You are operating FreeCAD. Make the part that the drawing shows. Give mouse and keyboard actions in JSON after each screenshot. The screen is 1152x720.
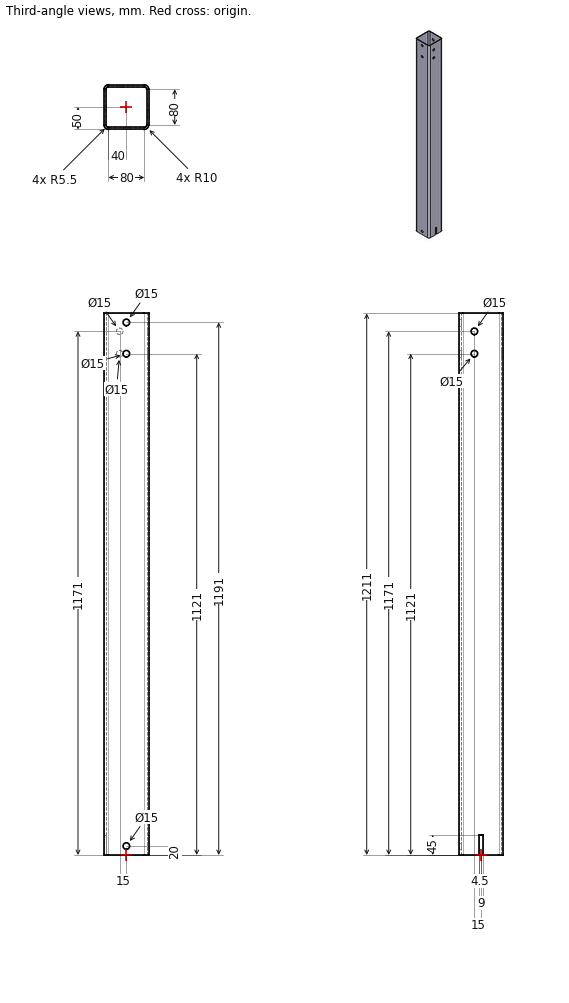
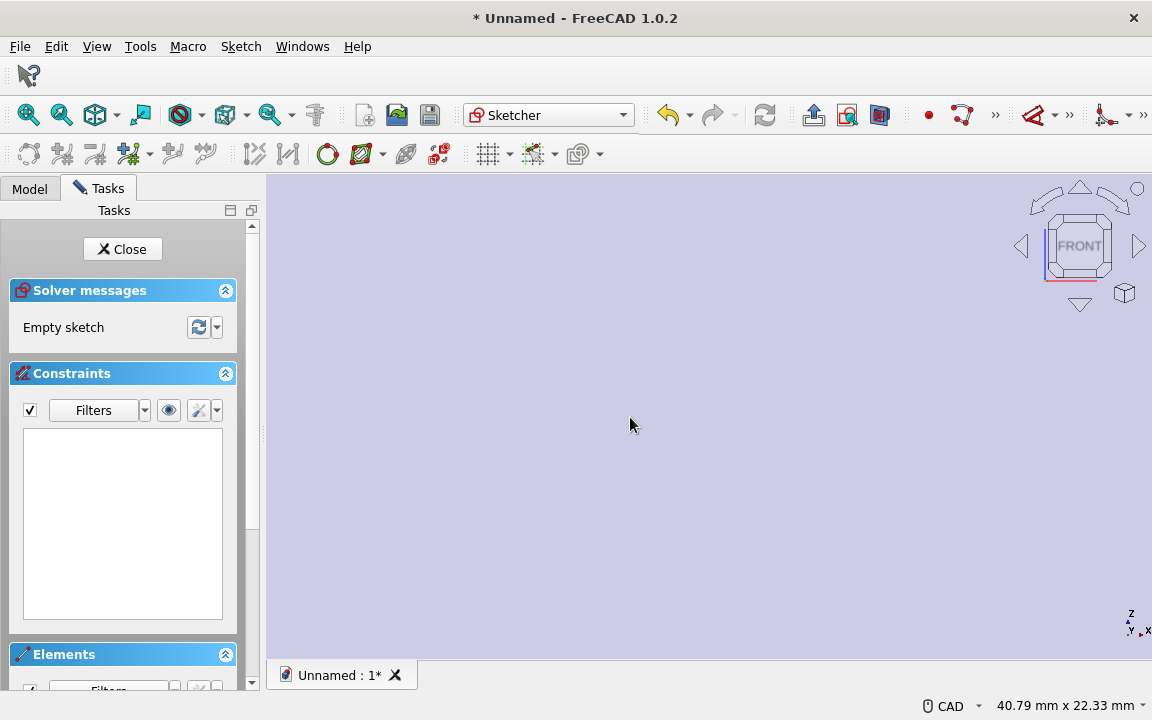
{"action": "key", "text": "g c"}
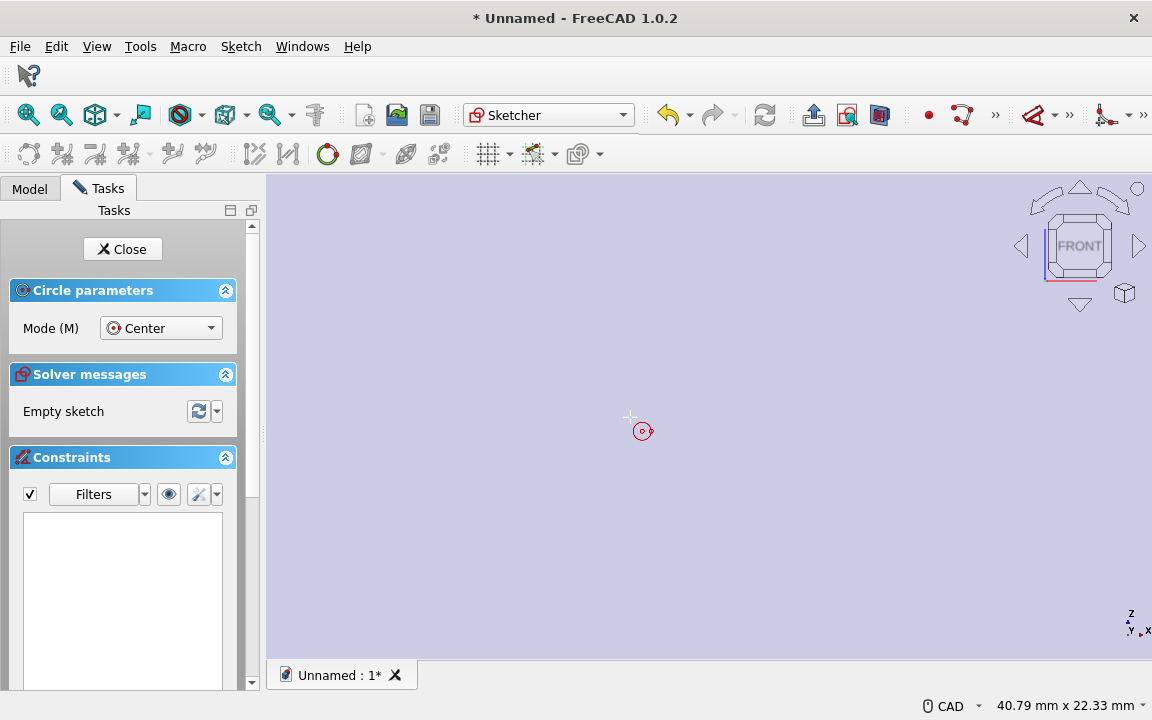
{"action": "left_click", "coordinate": [637, 412]}
{"action": "left_click", "coordinate": [752, 297]}
{"action": "key", "text": "Escape"}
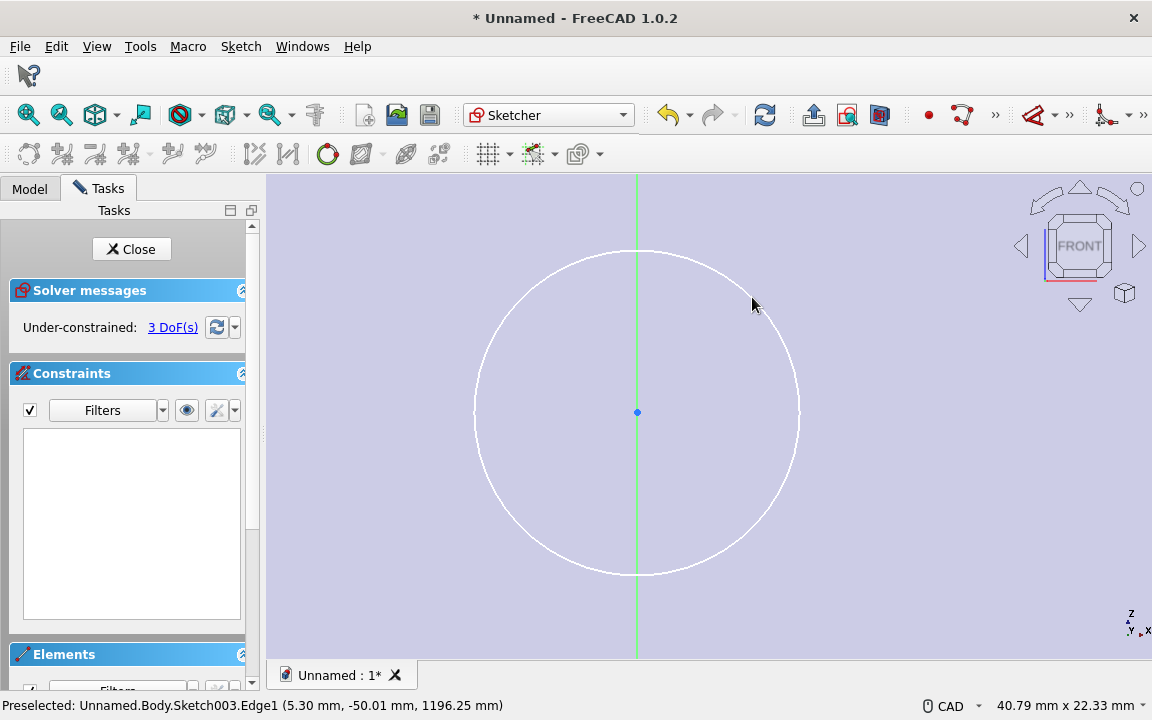
{"action": "left_click", "coordinate": [637, 413]}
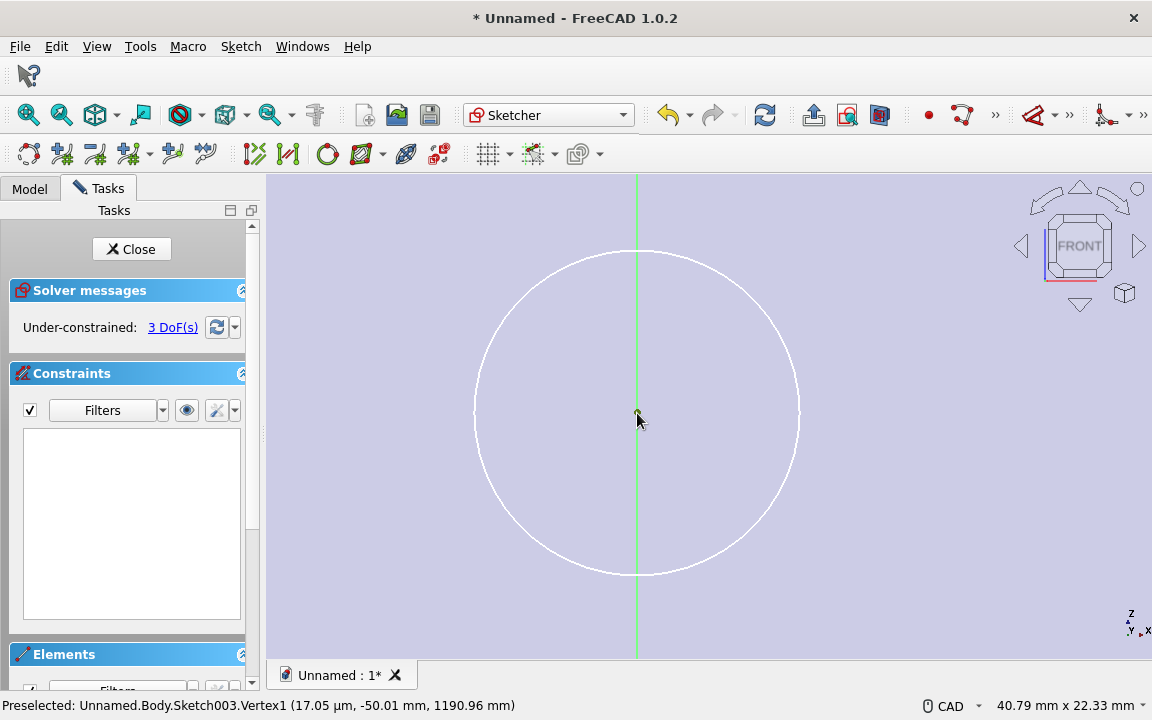
{"action": "left_click", "coordinate": [637, 539]}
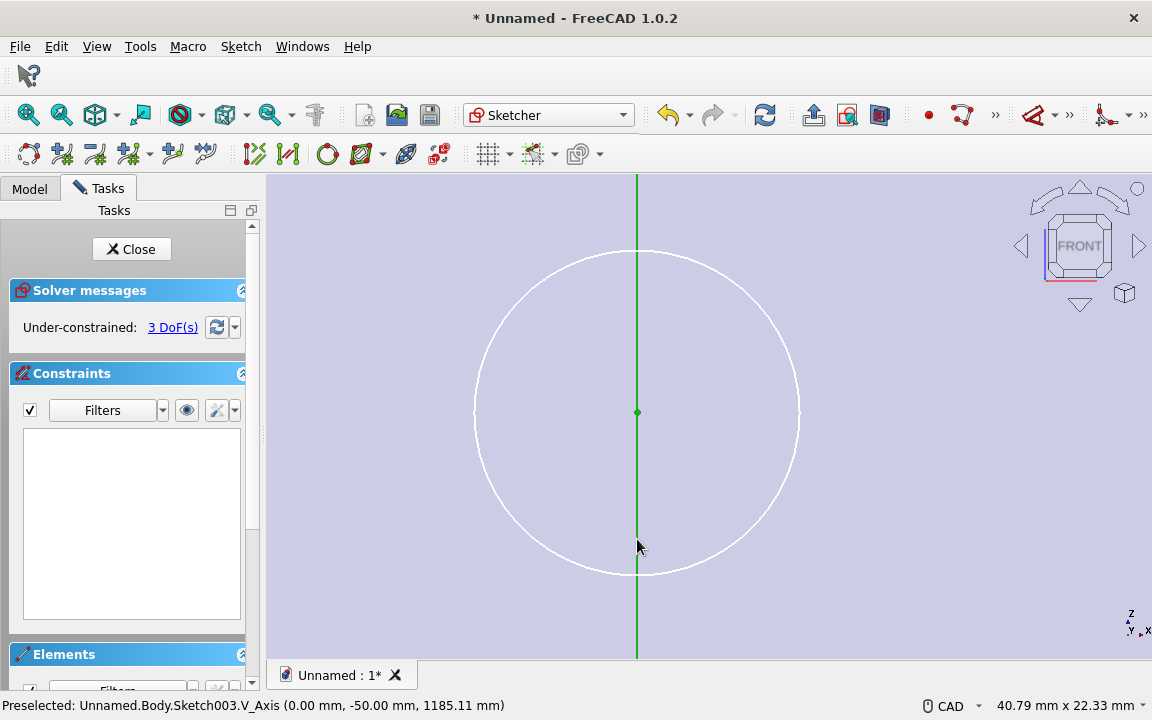
{"action": "key", "text": "c"}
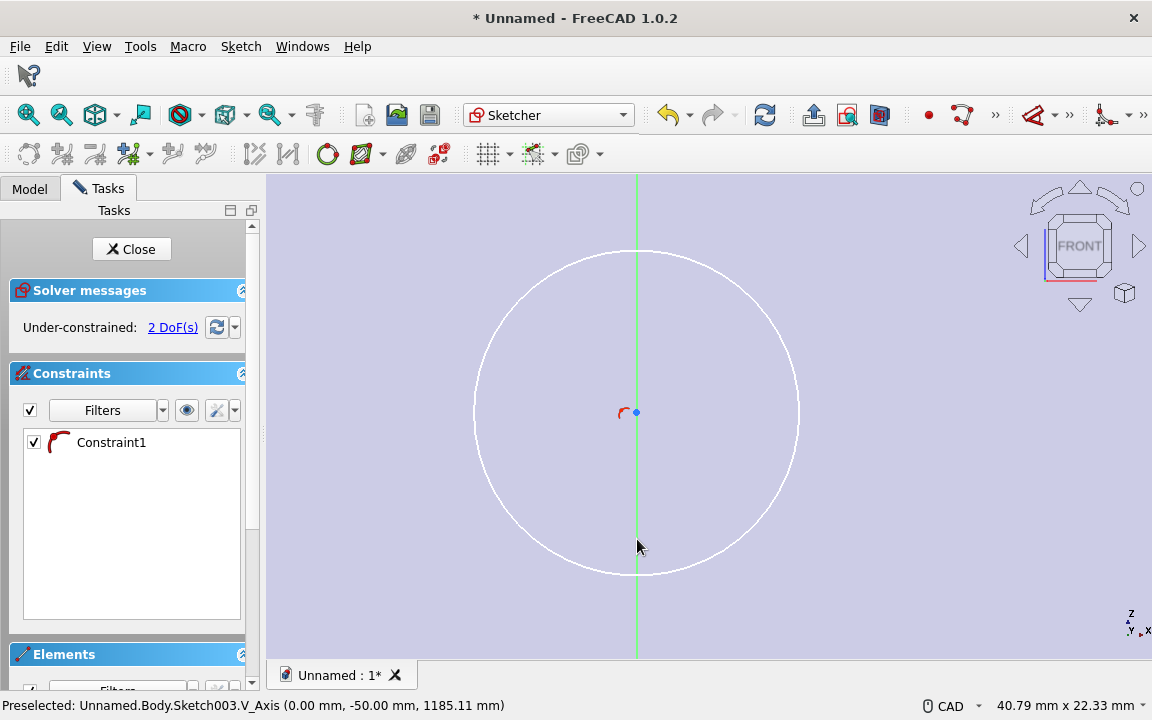
{"action": "key", "text": "d"}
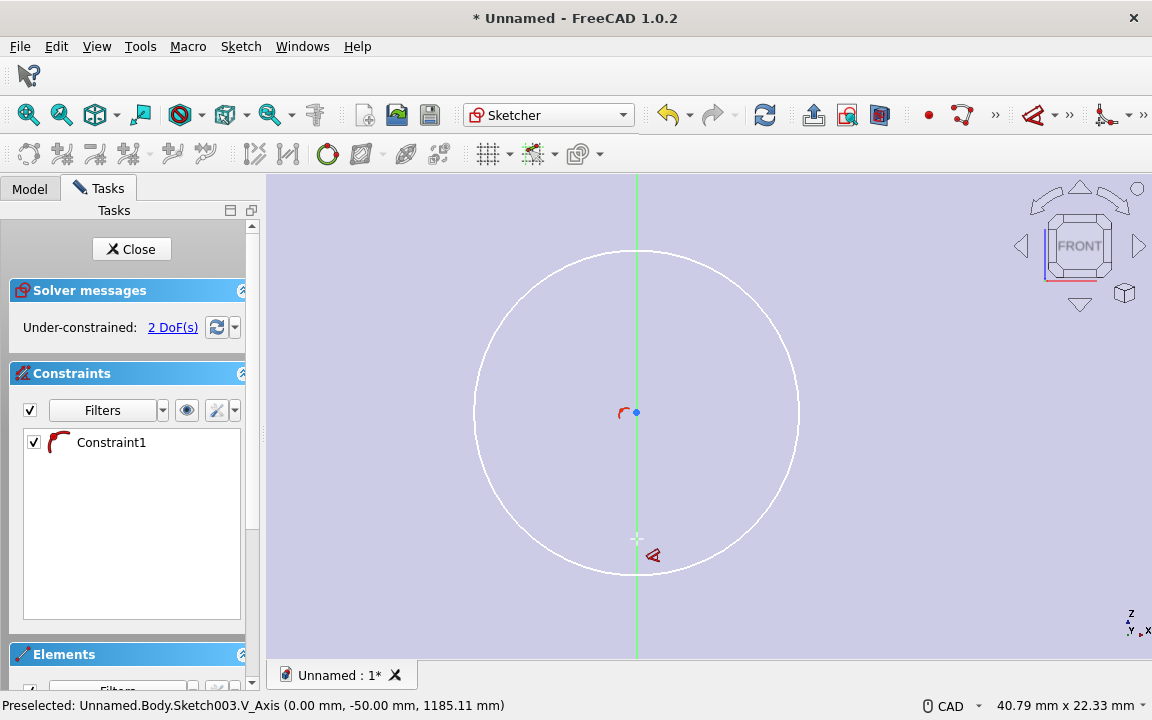
{"action": "left_click", "coordinate": [751, 298]}
{"action": "left_click", "coordinate": [774, 275]}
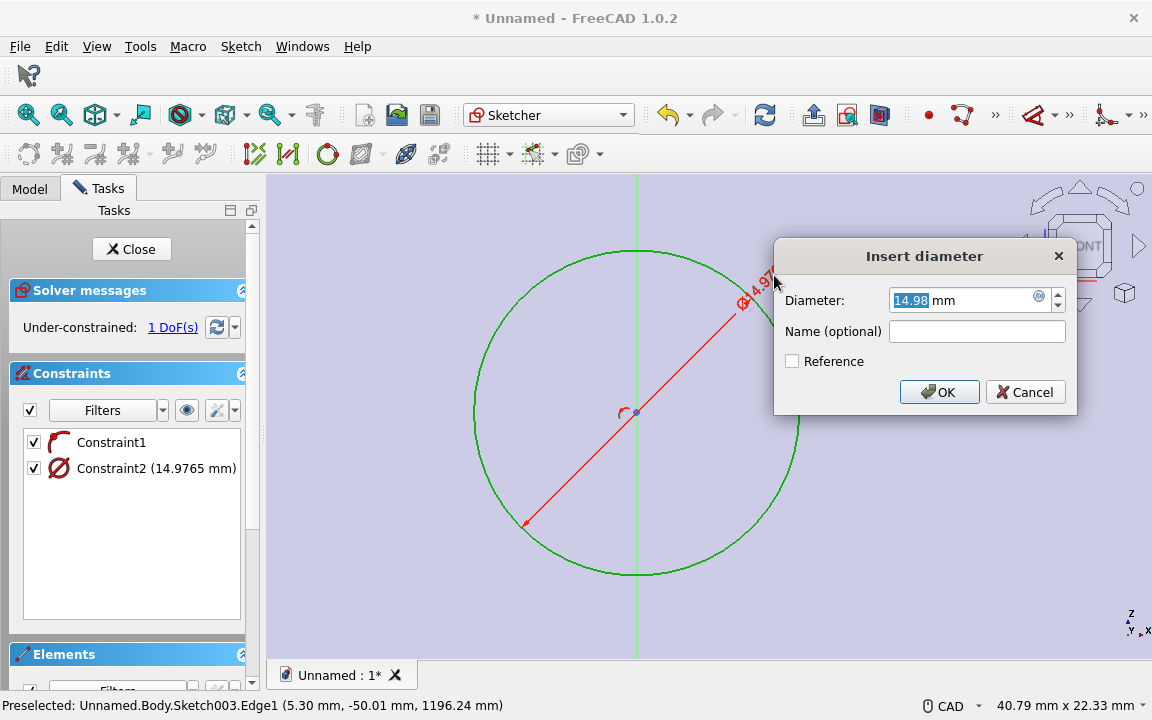
{"action": "type", "text": "15"}
{"action": "key", "text": "Return"}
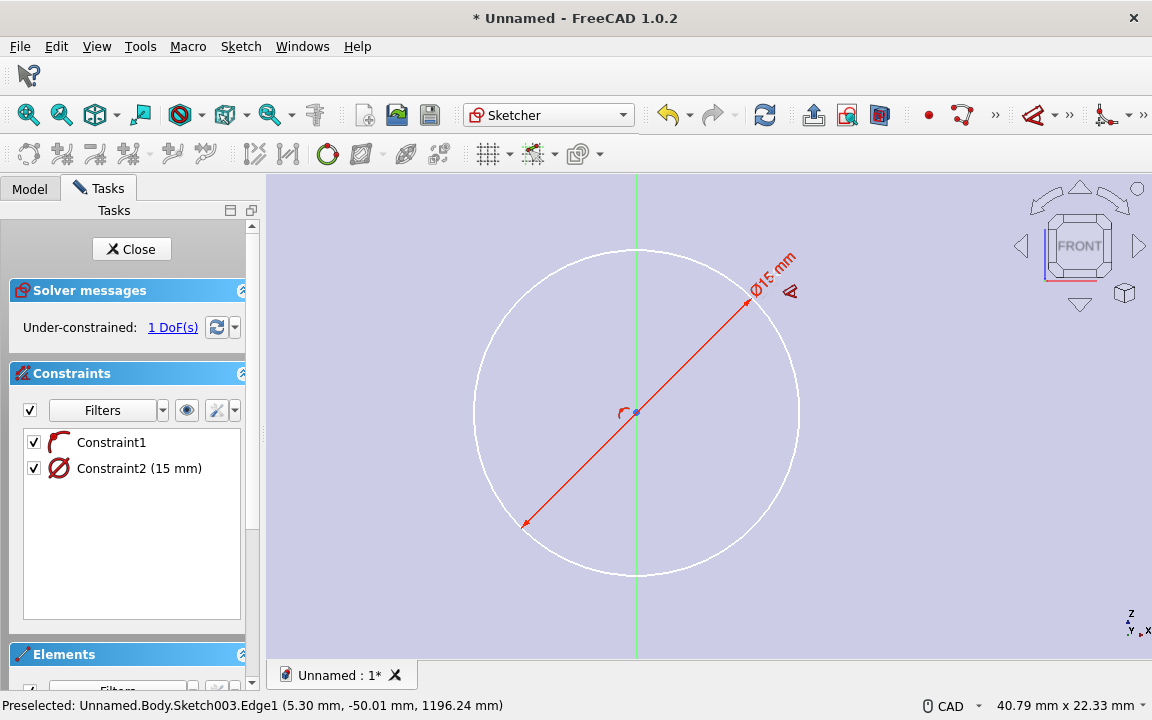
{"action": "left_click", "coordinate": [637, 413]}
{"action": "left_click", "coordinate": [671, 522]}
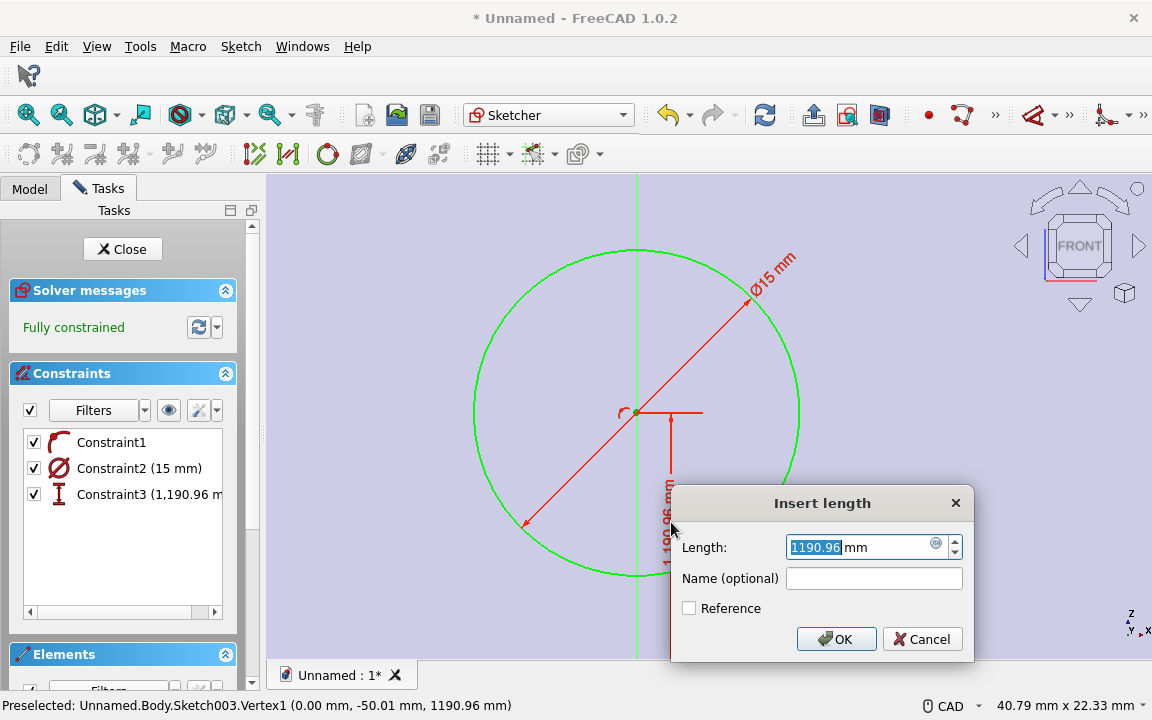
{"action": "type", "text": "1191"}
{"action": "key", "text": "Return"}
{"action": "key", "text": "Escape"}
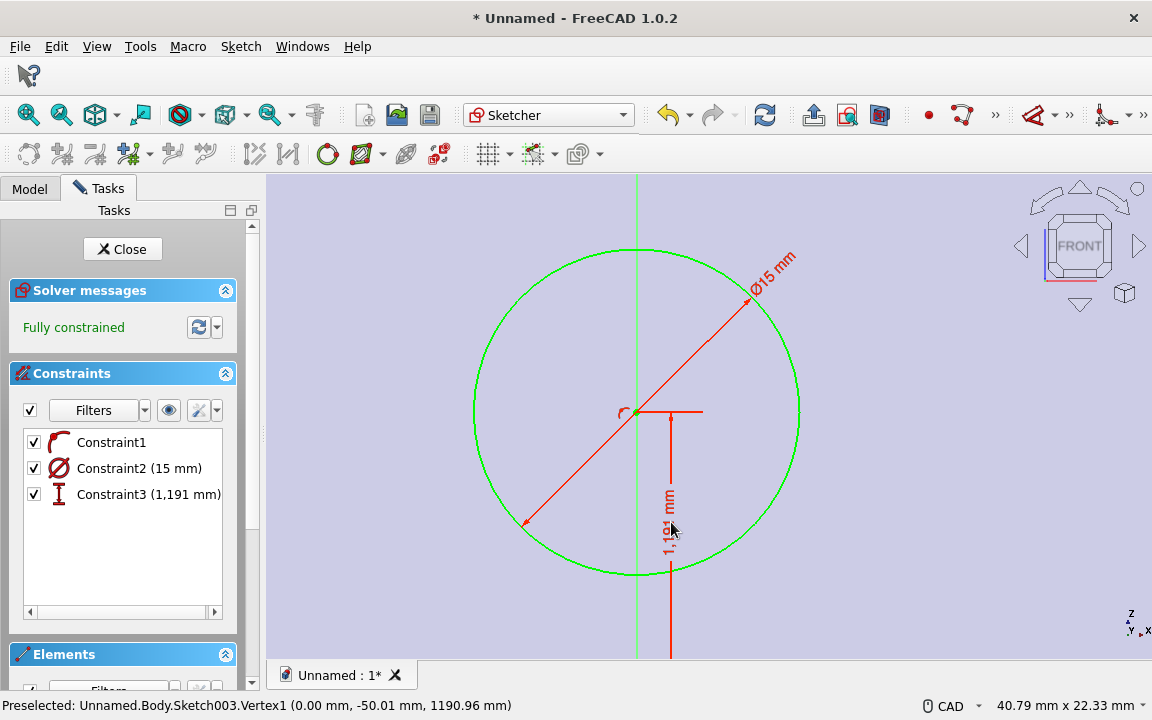
{"action": "left_click", "coordinate": [123, 249]}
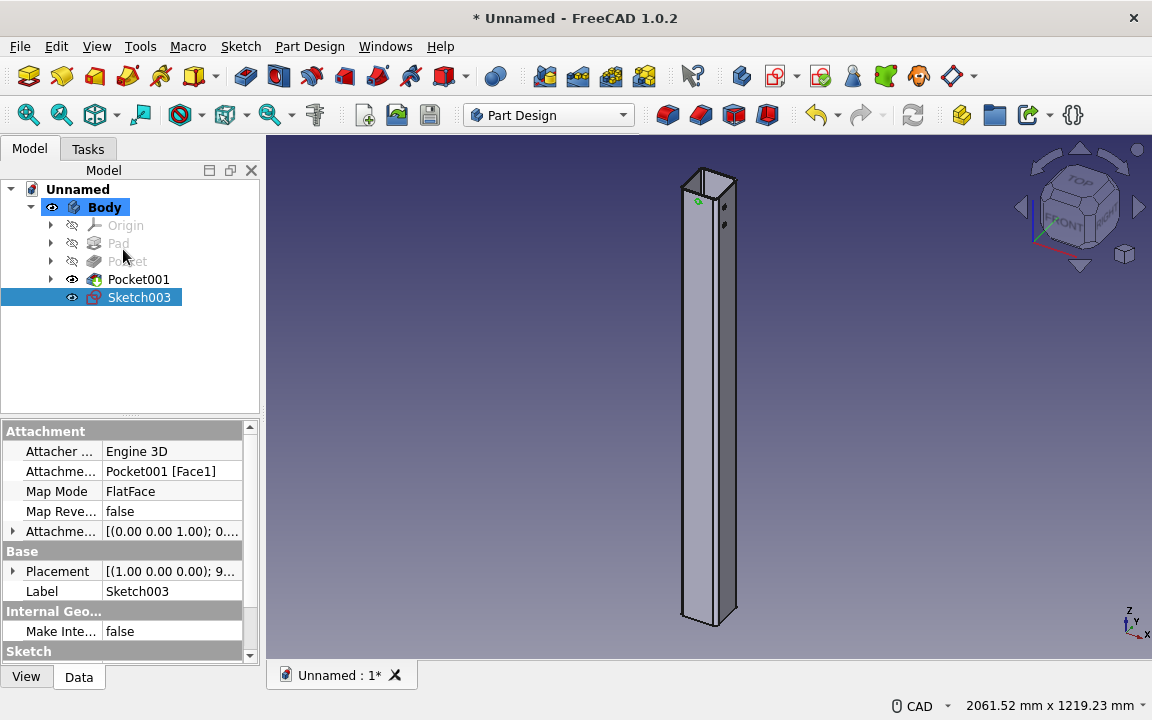
{"action": "left_click", "coordinate": [246, 76]}